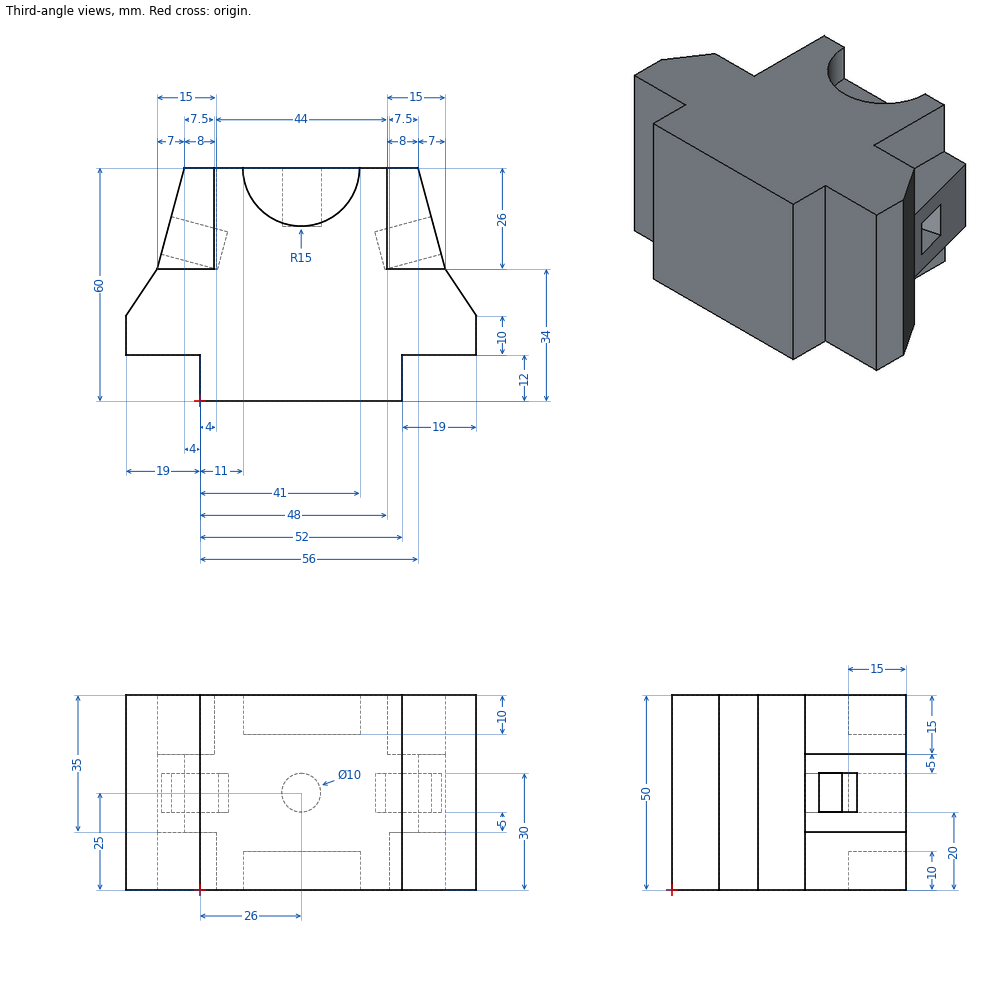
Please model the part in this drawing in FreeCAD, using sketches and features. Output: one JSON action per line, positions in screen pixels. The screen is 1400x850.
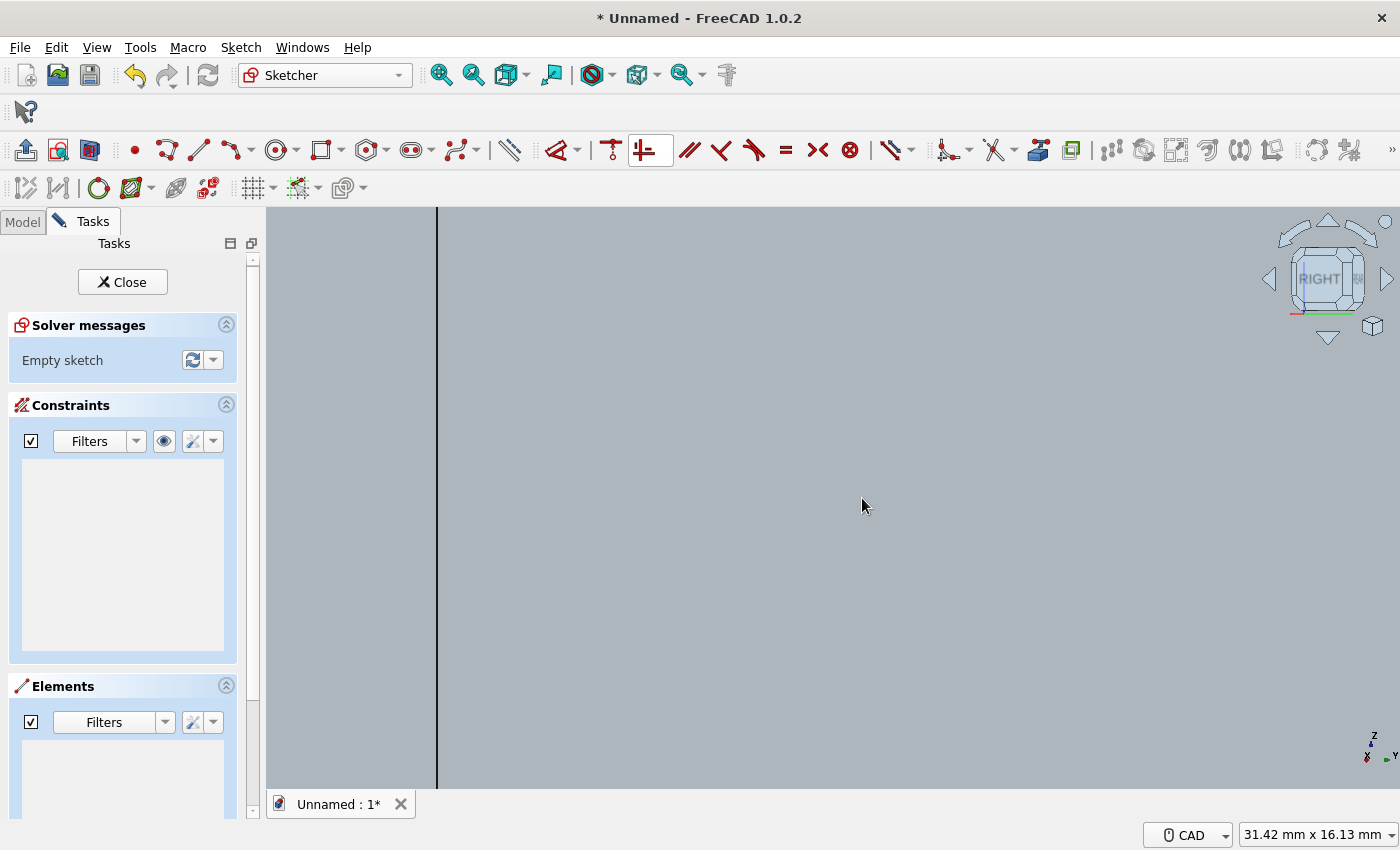
{"action": "left_click", "coordinate": [322, 150]}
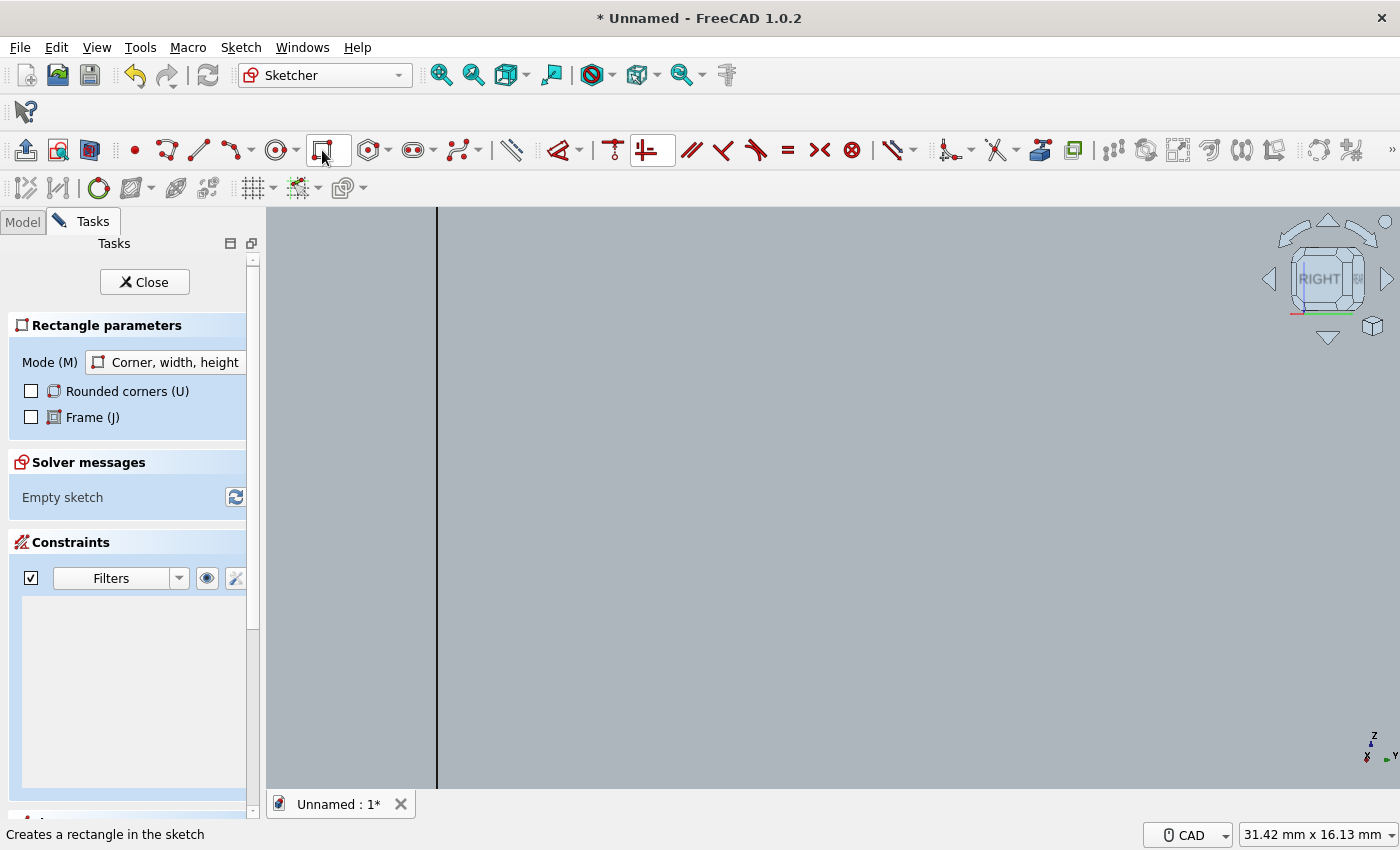
{"action": "left_click", "coordinate": [578, 314]}
{"action": "left_click", "coordinate": [939, 675]}
{"action": "key", "text": "Escape"}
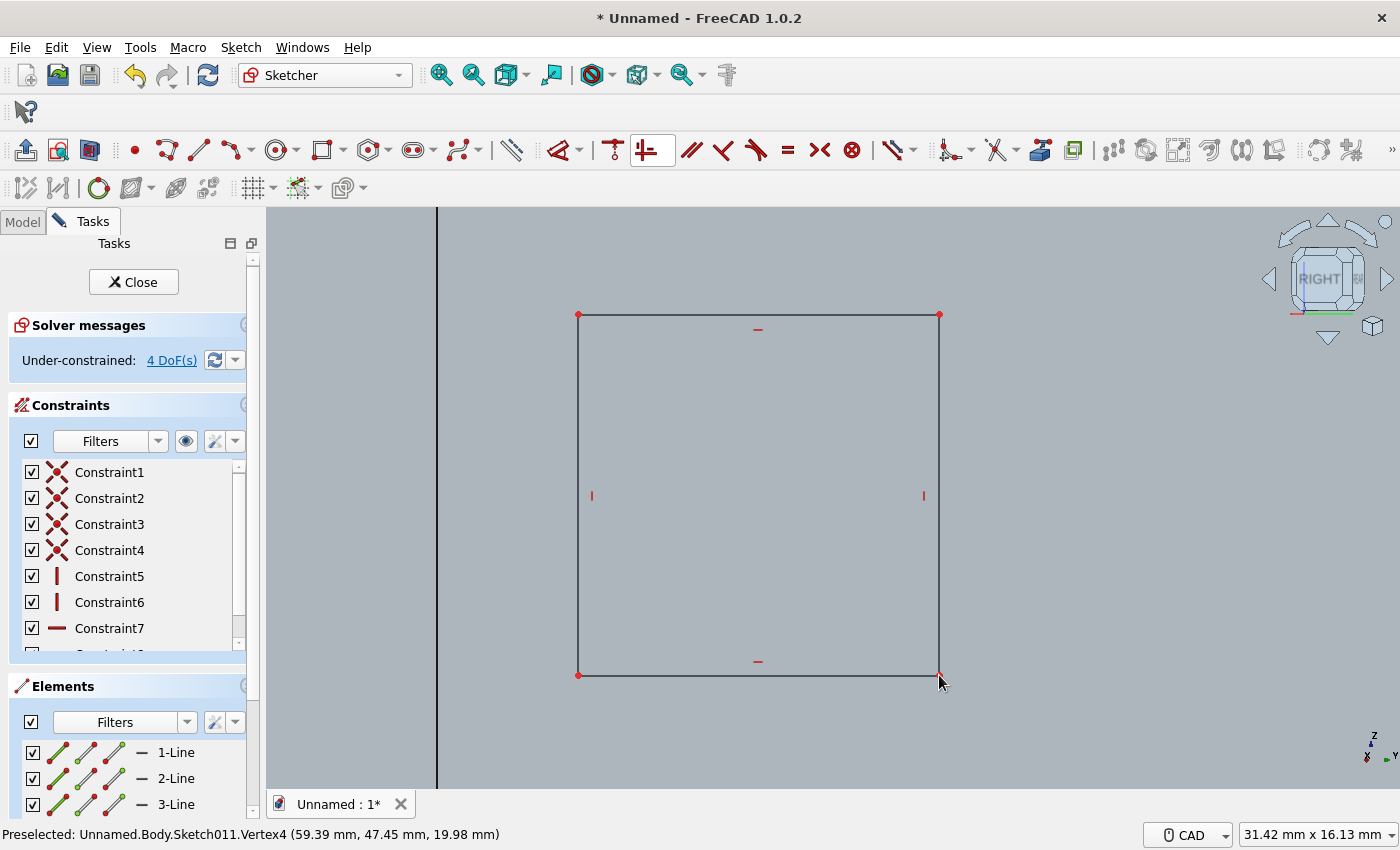
{"action": "left_click", "coordinate": [558, 150]}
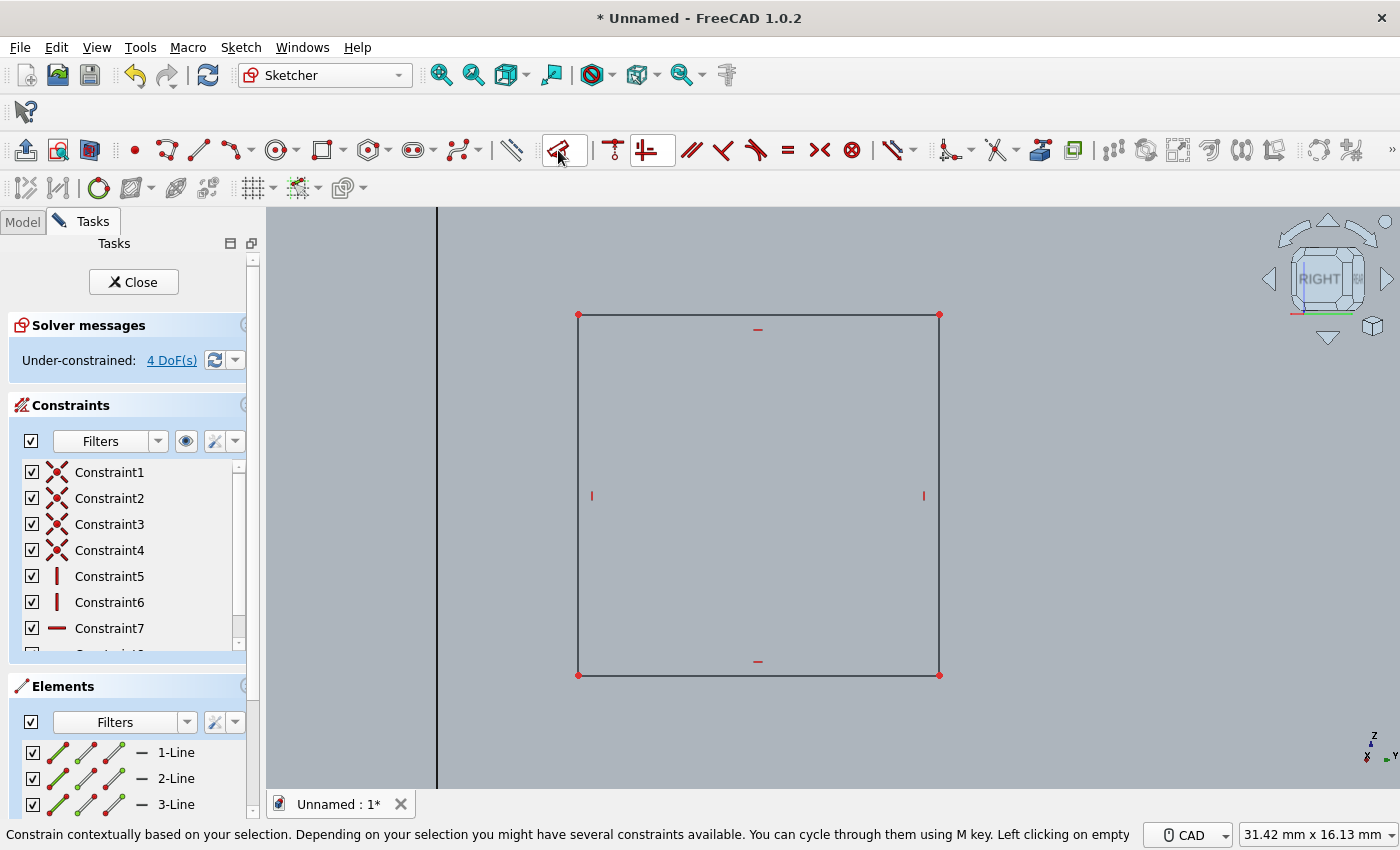
{"action": "left_click", "coordinate": [578, 423]}
{"action": "left_click", "coordinate": [544, 495]}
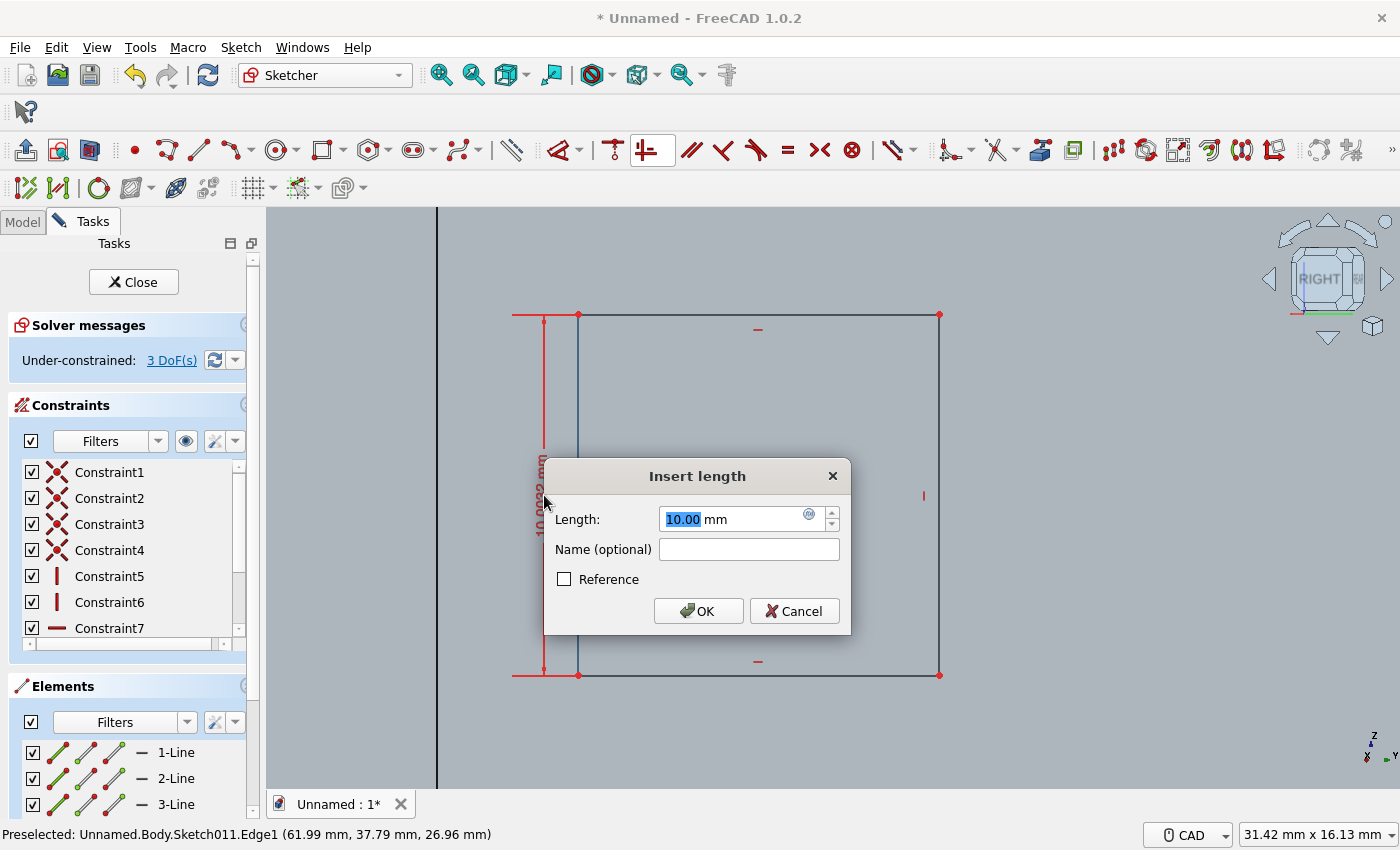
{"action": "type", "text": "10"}
{"action": "key", "text": "Return"}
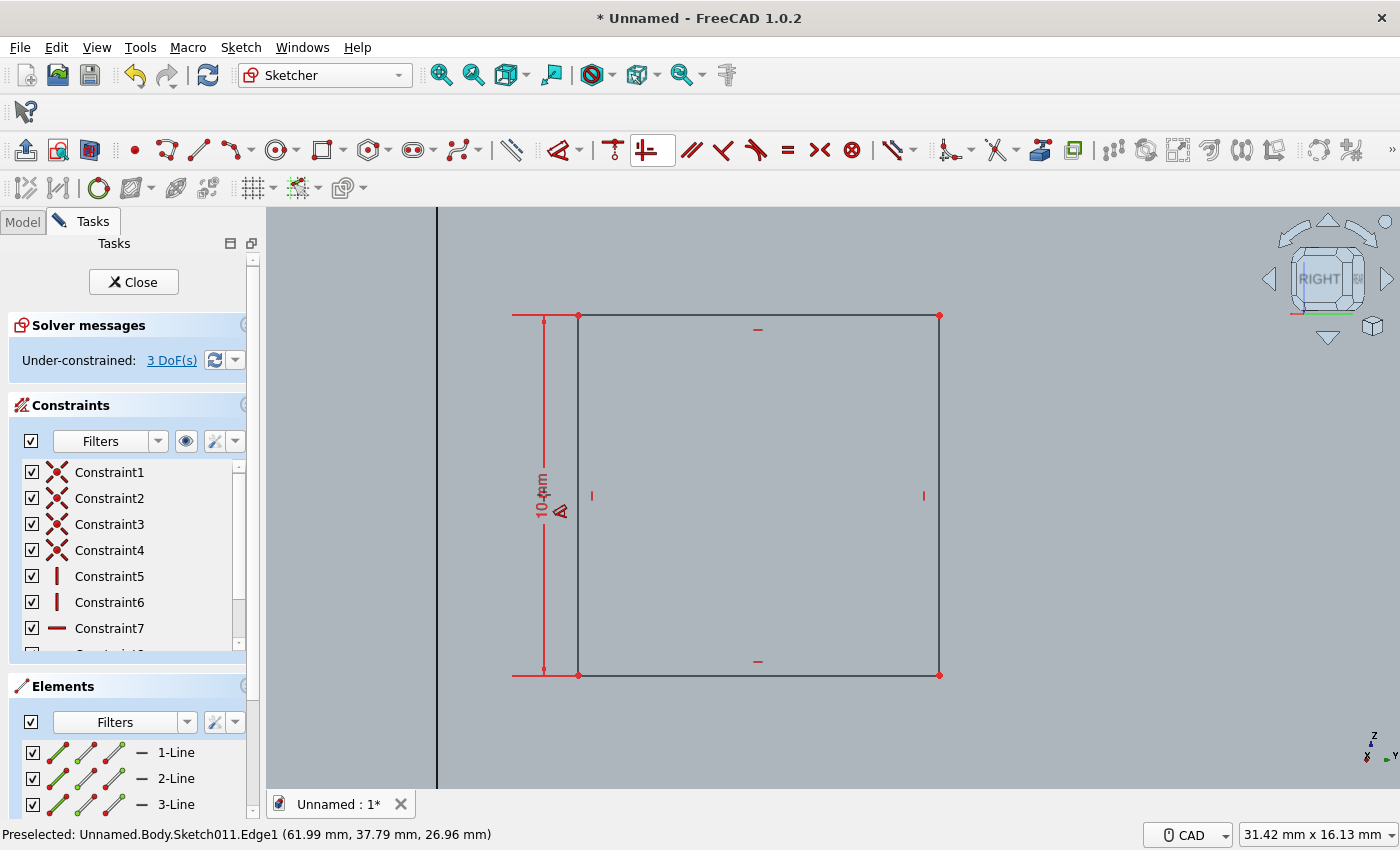
{"action": "left_click", "coordinate": [686, 676]}
{"action": "left_click", "coordinate": [759, 710]}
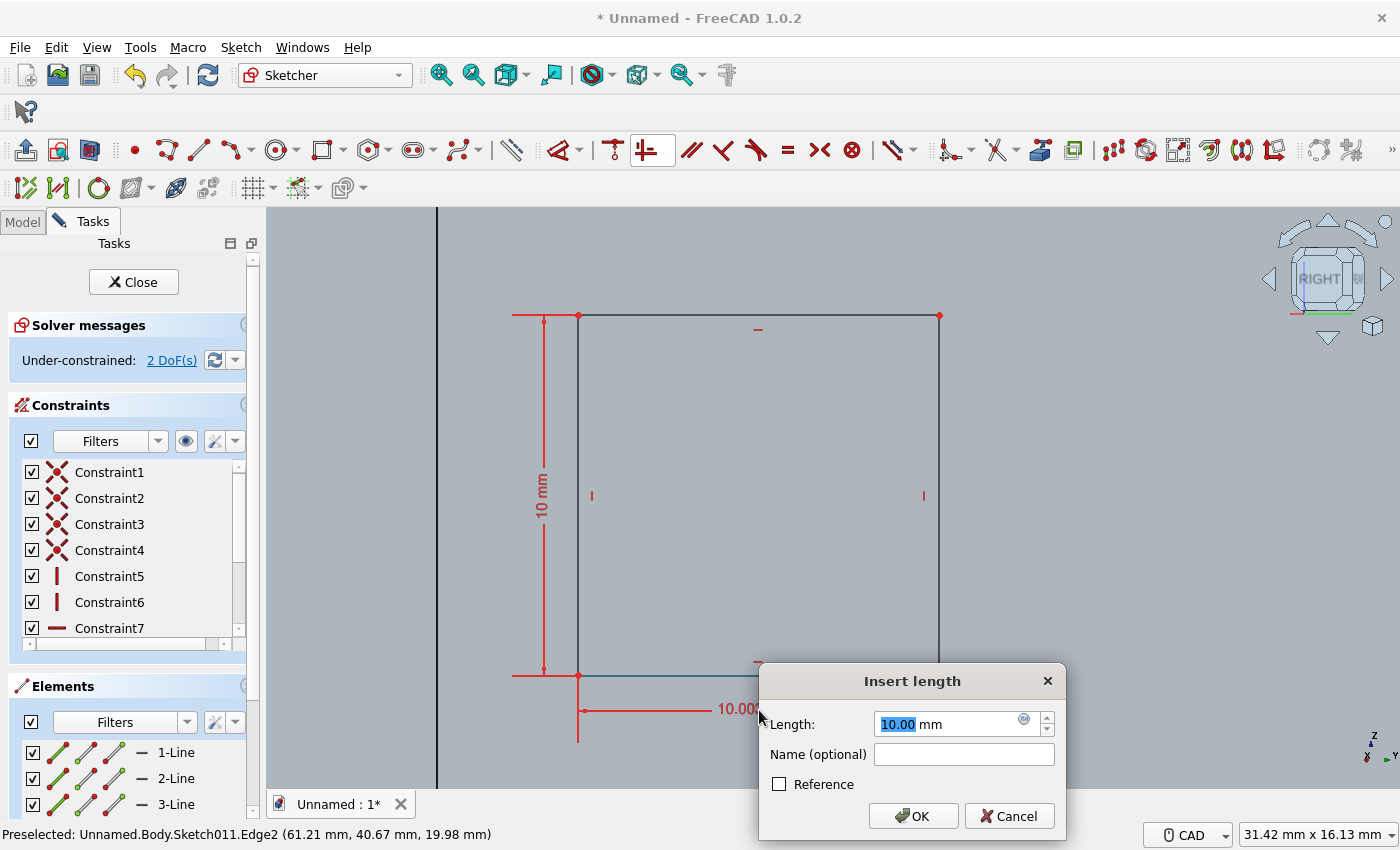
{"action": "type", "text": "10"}
{"action": "key", "text": "Return"}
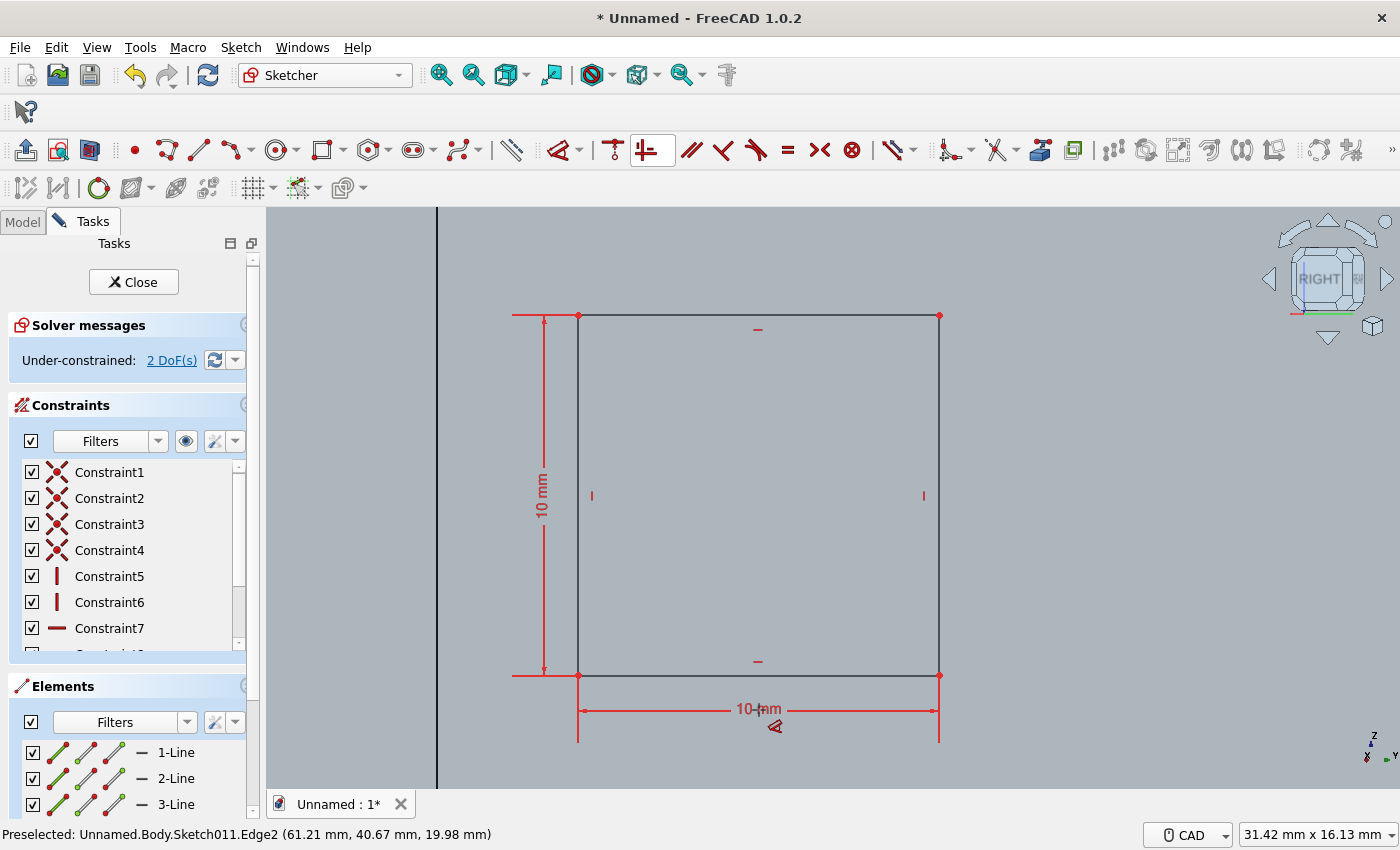
{"action": "left_click", "coordinate": [578, 315]}
{"action": "left_click", "coordinate": [612, 538]}